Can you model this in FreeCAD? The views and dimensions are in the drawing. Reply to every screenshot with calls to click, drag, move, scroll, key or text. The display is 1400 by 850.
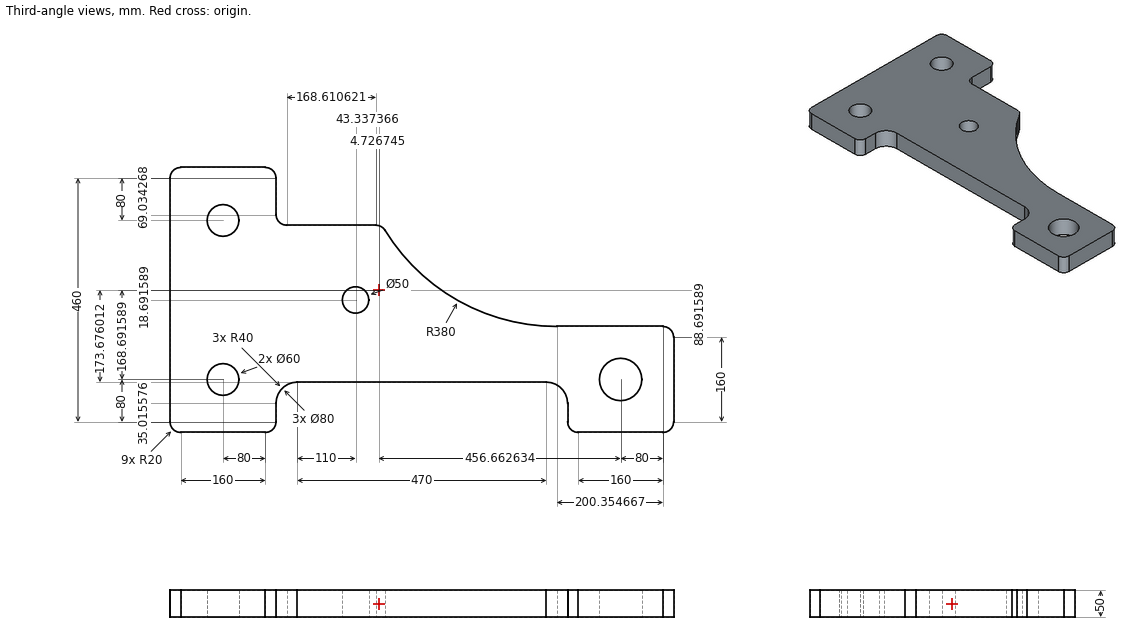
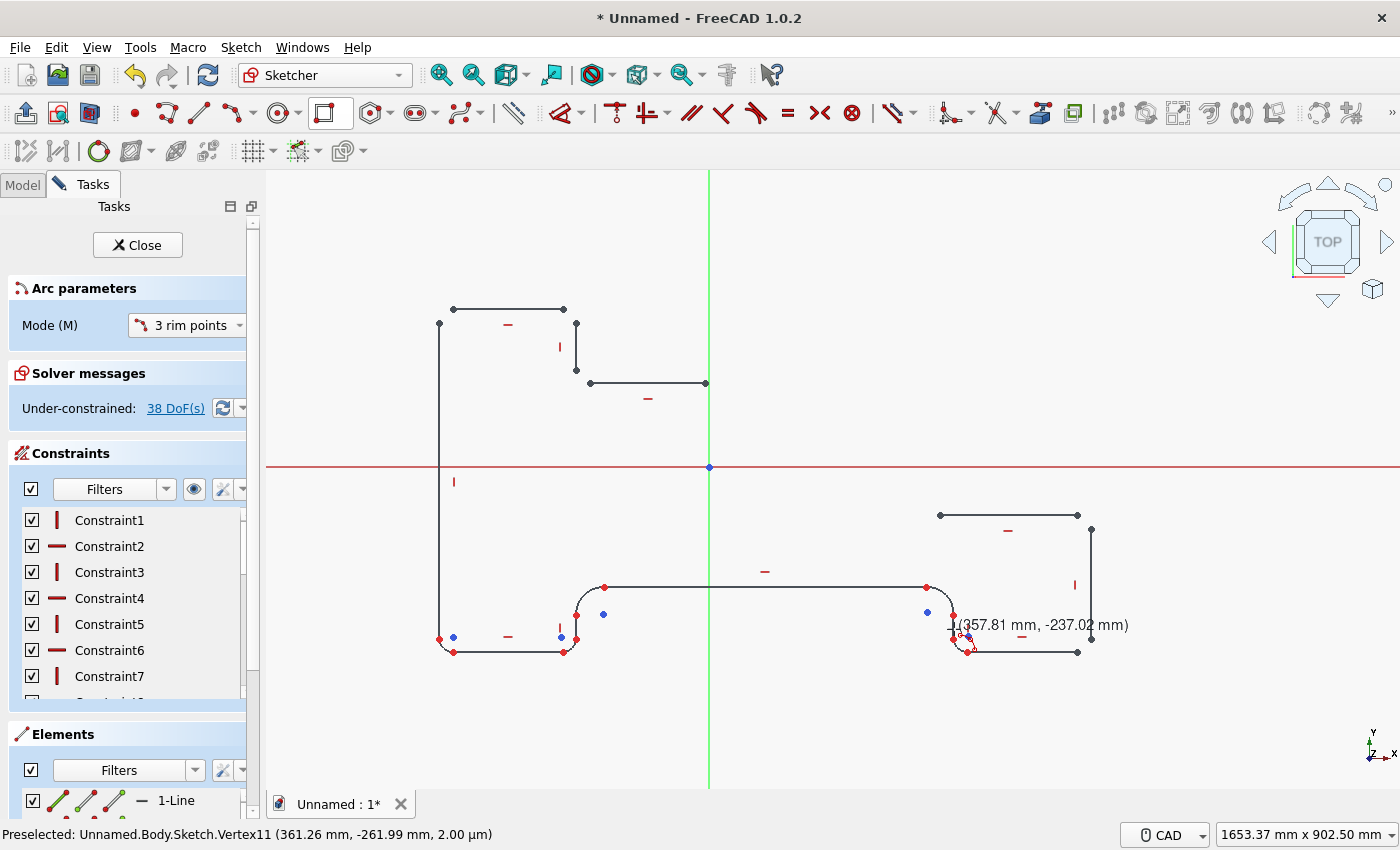
click(1077, 652)
click(1091, 639)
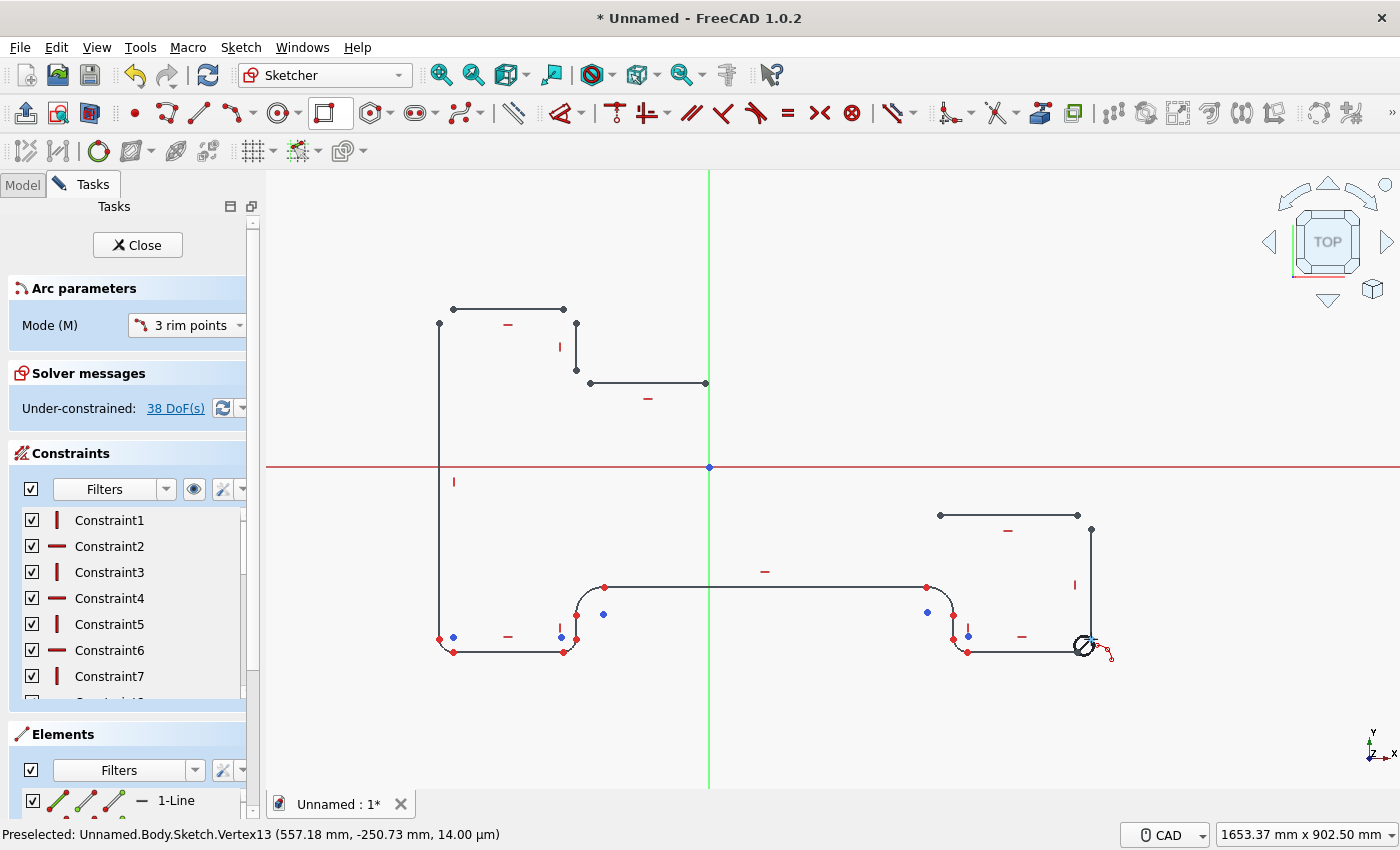
scroll(1087, 648, up, 7)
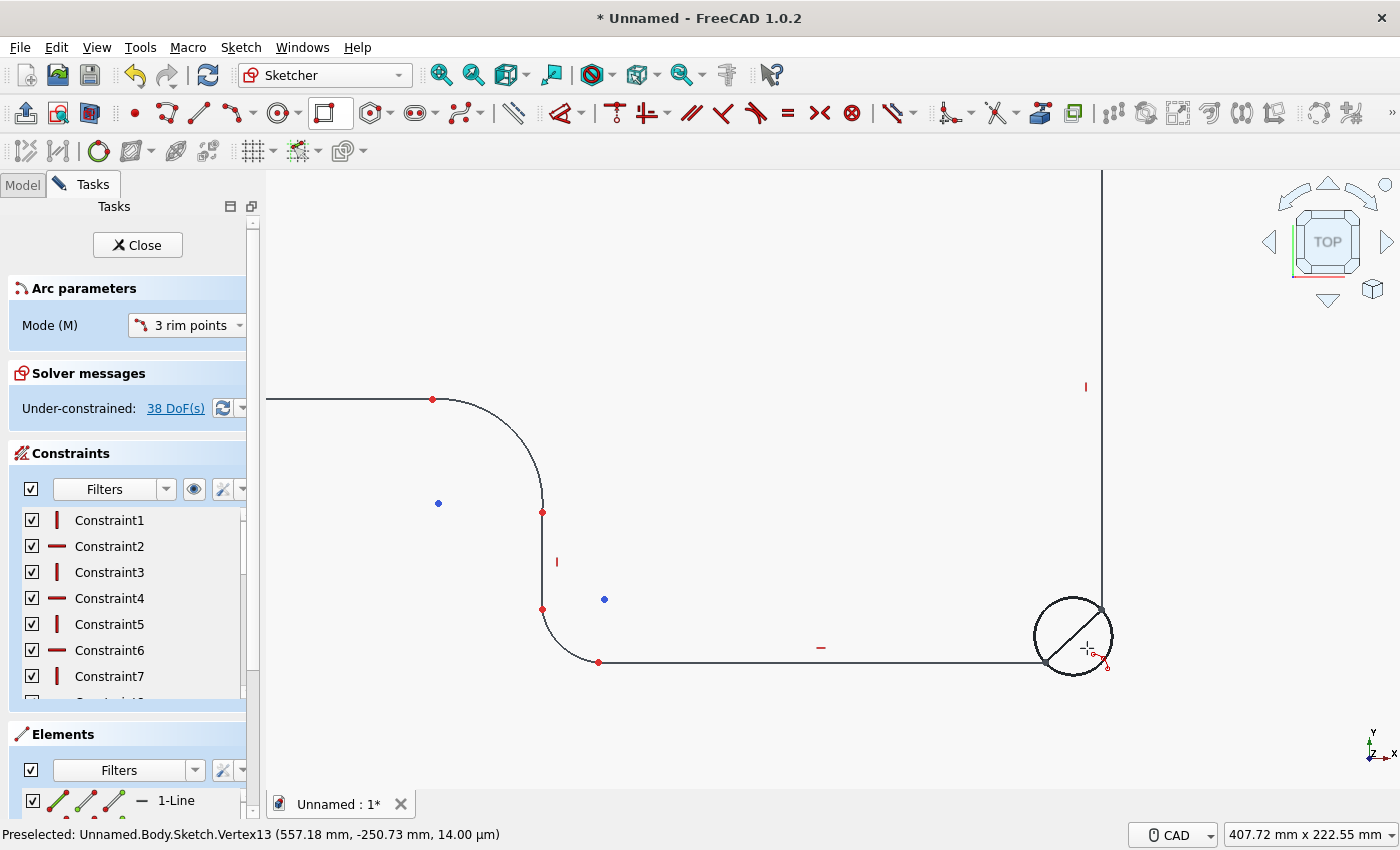
click(1084, 644)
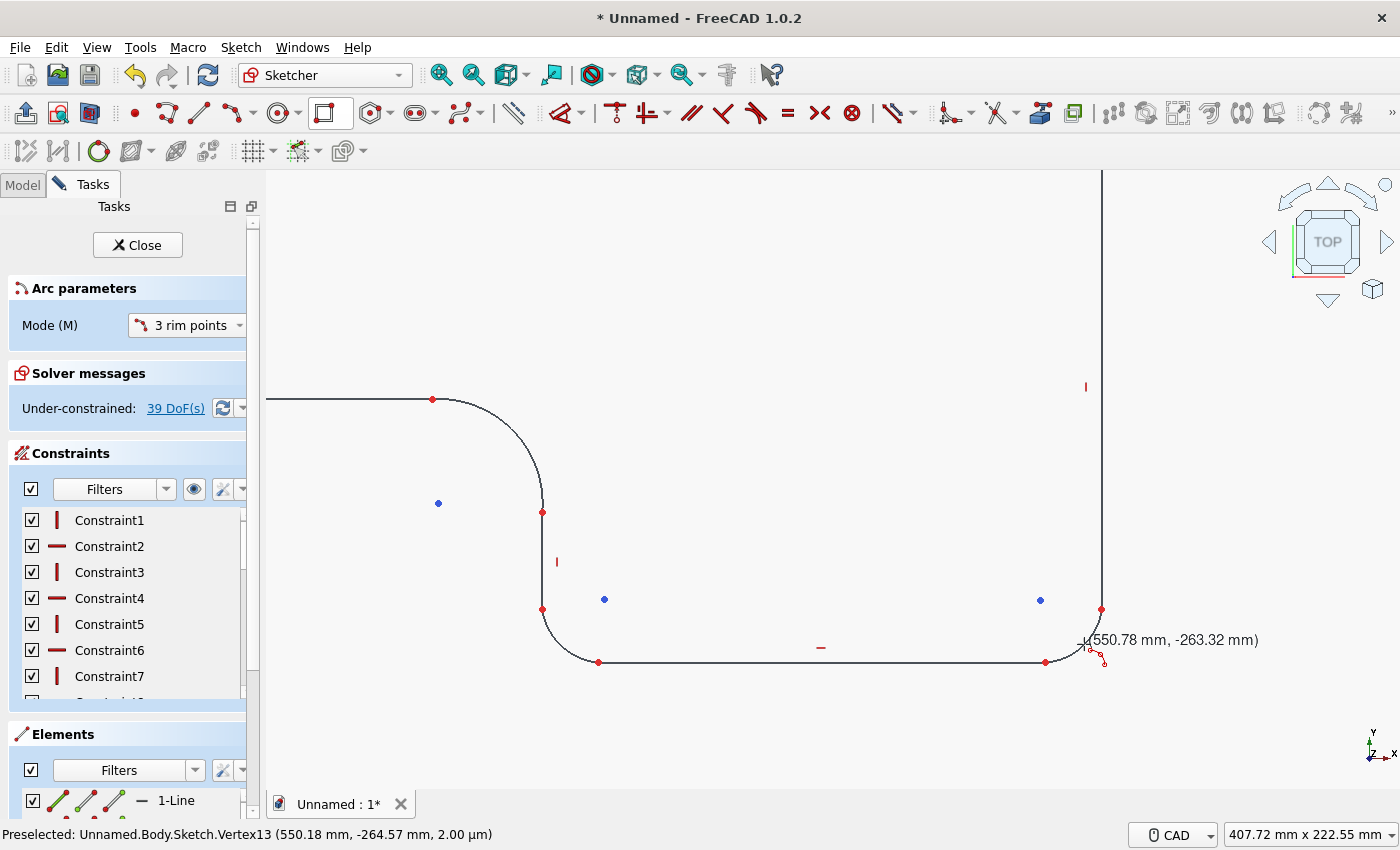
scroll(1087, 648, down, 7)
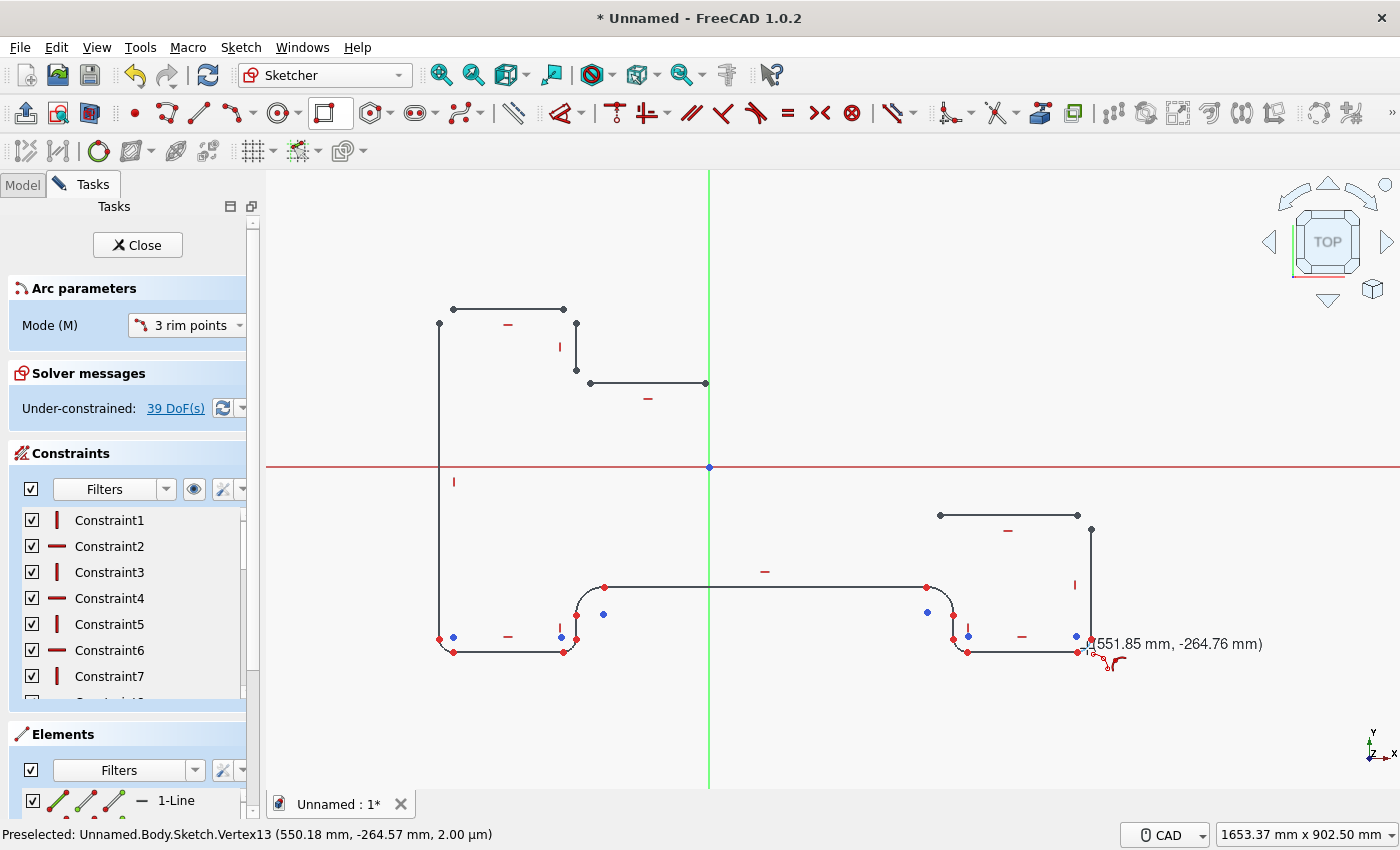
click(1091, 529)
click(1077, 515)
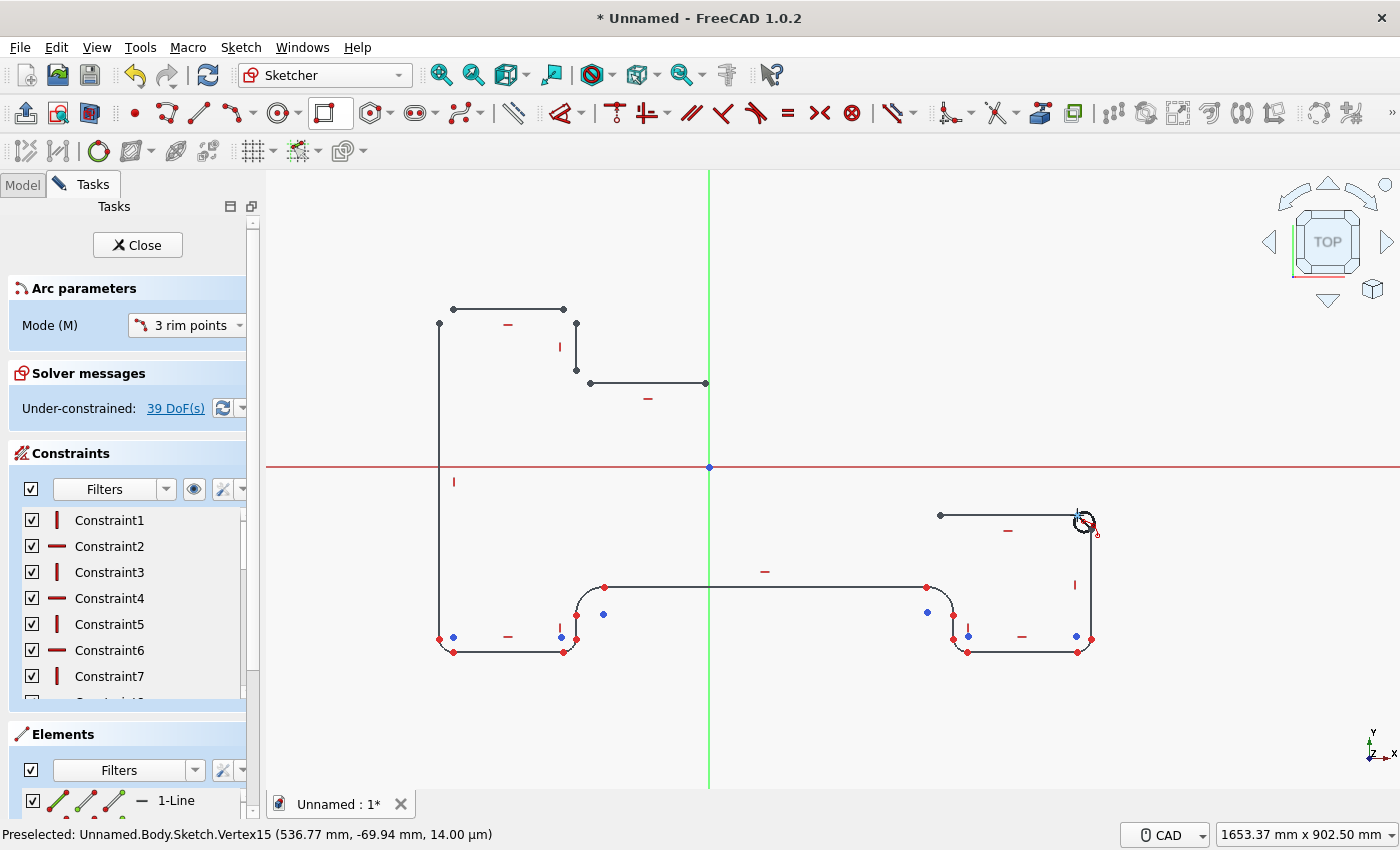
scroll(1087, 518, up, 7)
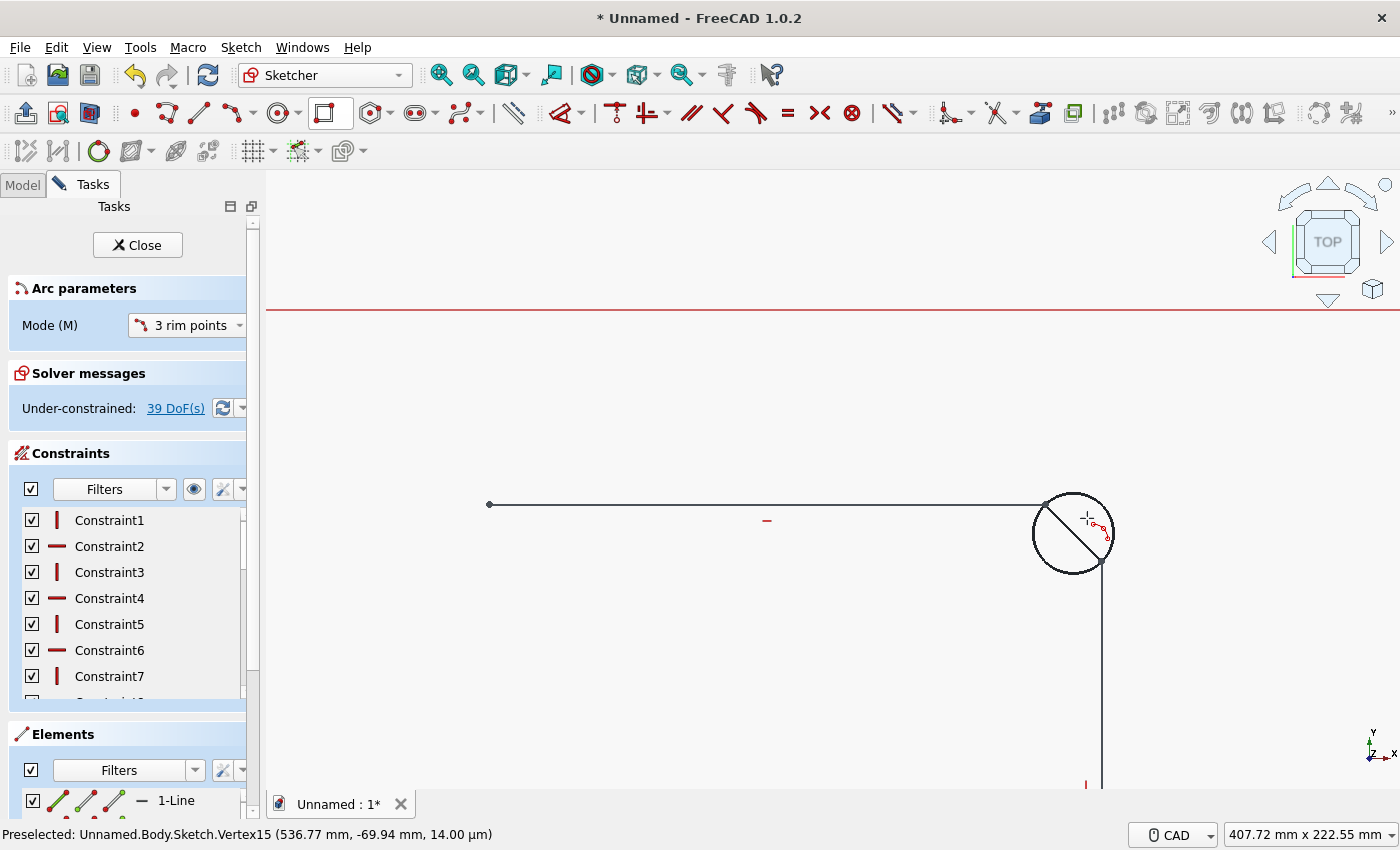
click(1084, 518)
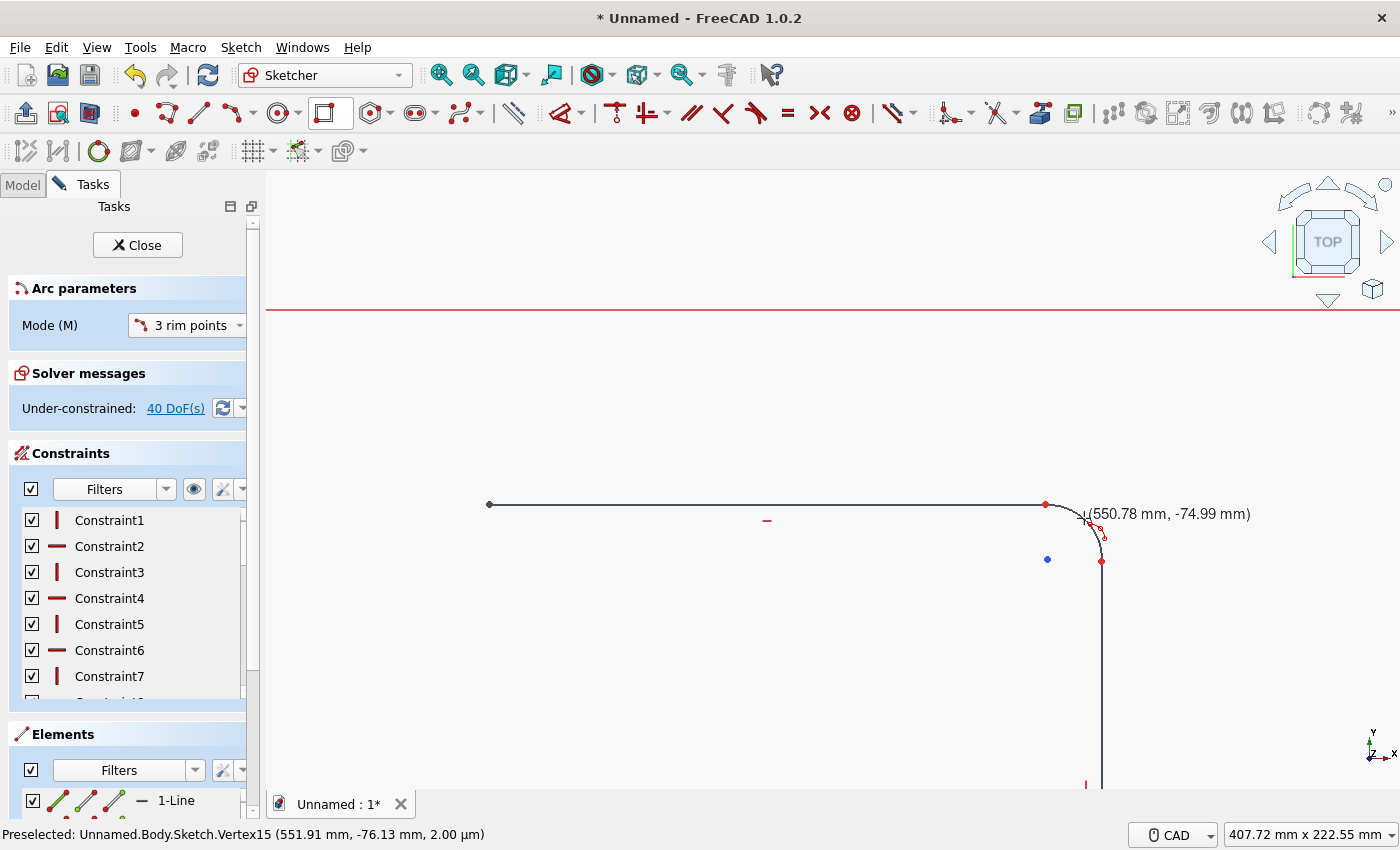
scroll(1087, 518, down, 7)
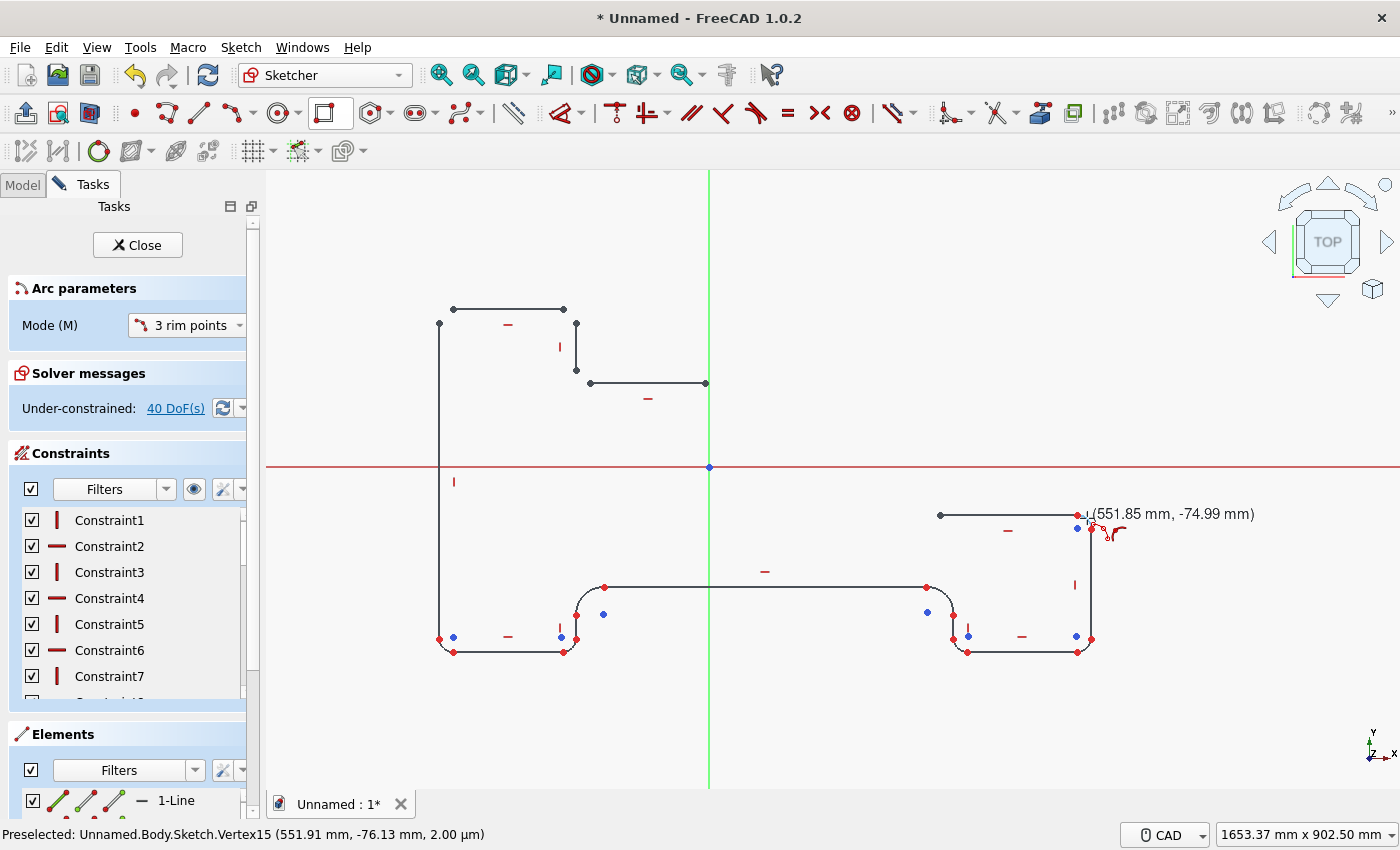
click(940, 515)